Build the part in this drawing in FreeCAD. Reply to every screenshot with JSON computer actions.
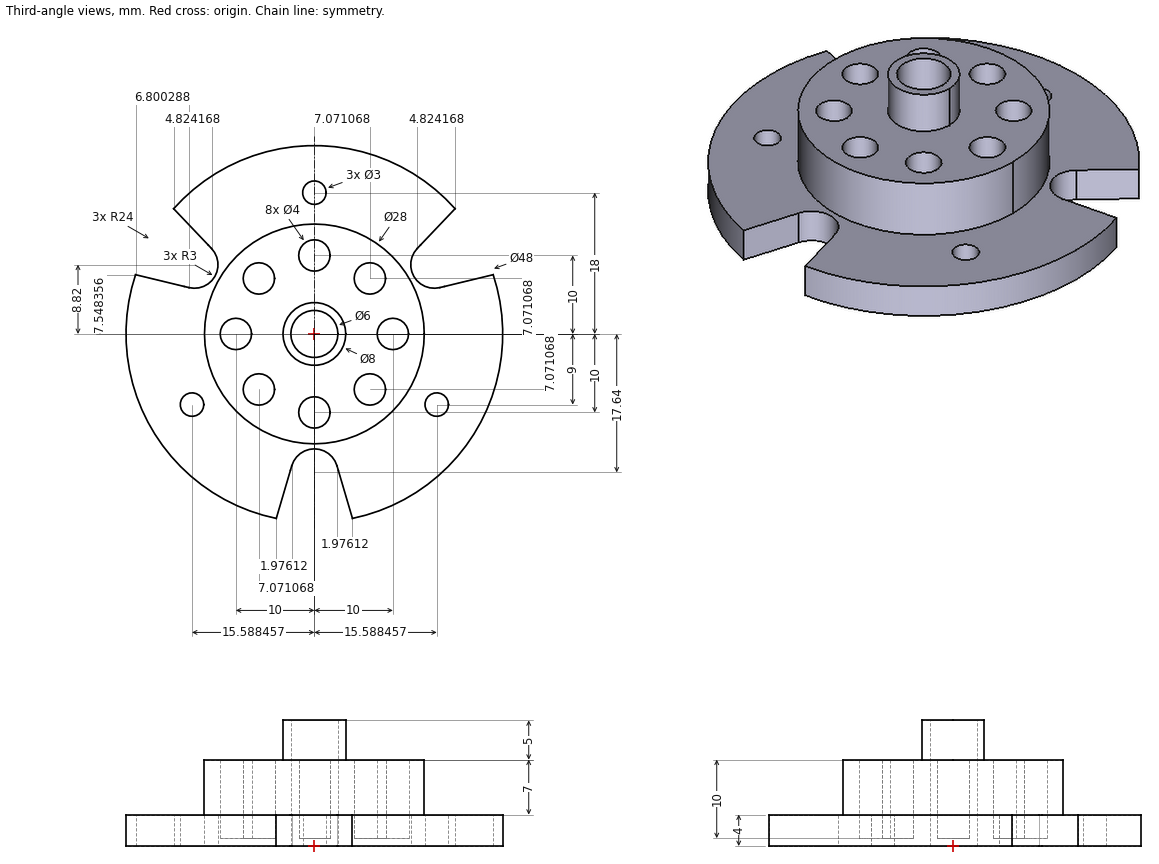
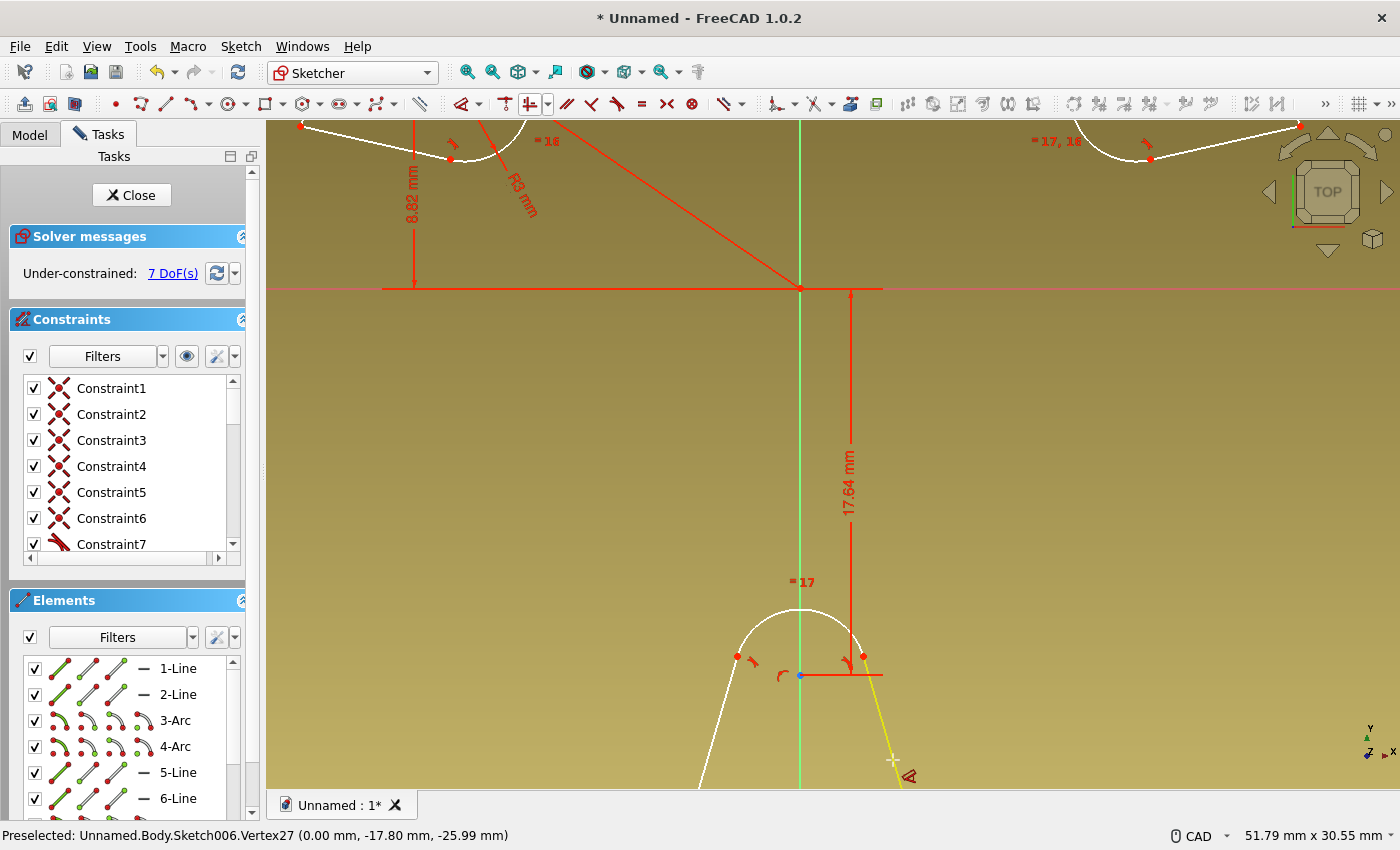
{"action": "left_click", "coordinate": [893, 760]}
{"action": "left_click", "coordinate": [885, 623]}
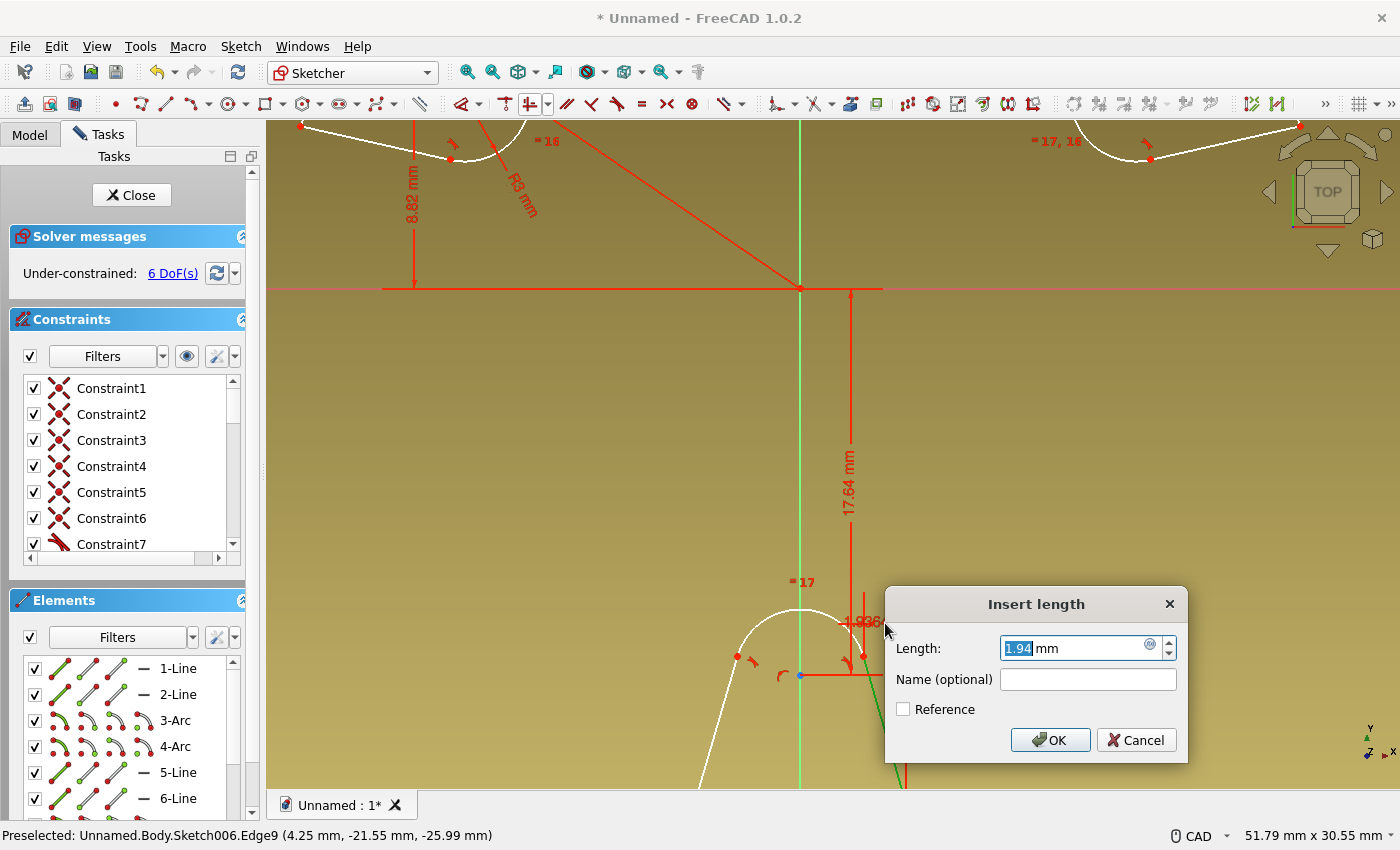
{"action": "type", "text": "1.97612"}
{"action": "key", "text": "Return"}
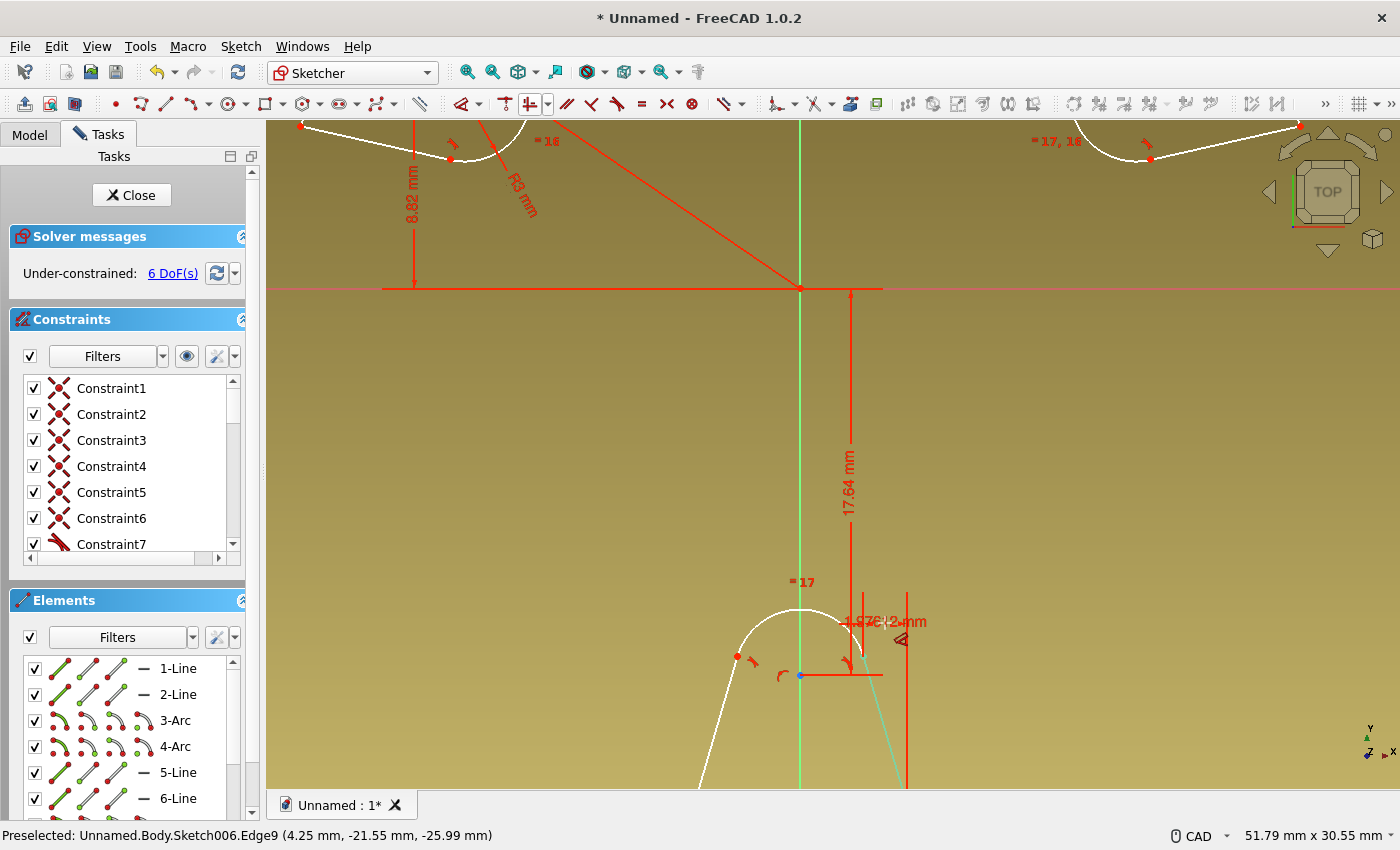
{"action": "left_click", "coordinate": [725, 701]}
{"action": "left_click", "coordinate": [716, 623]}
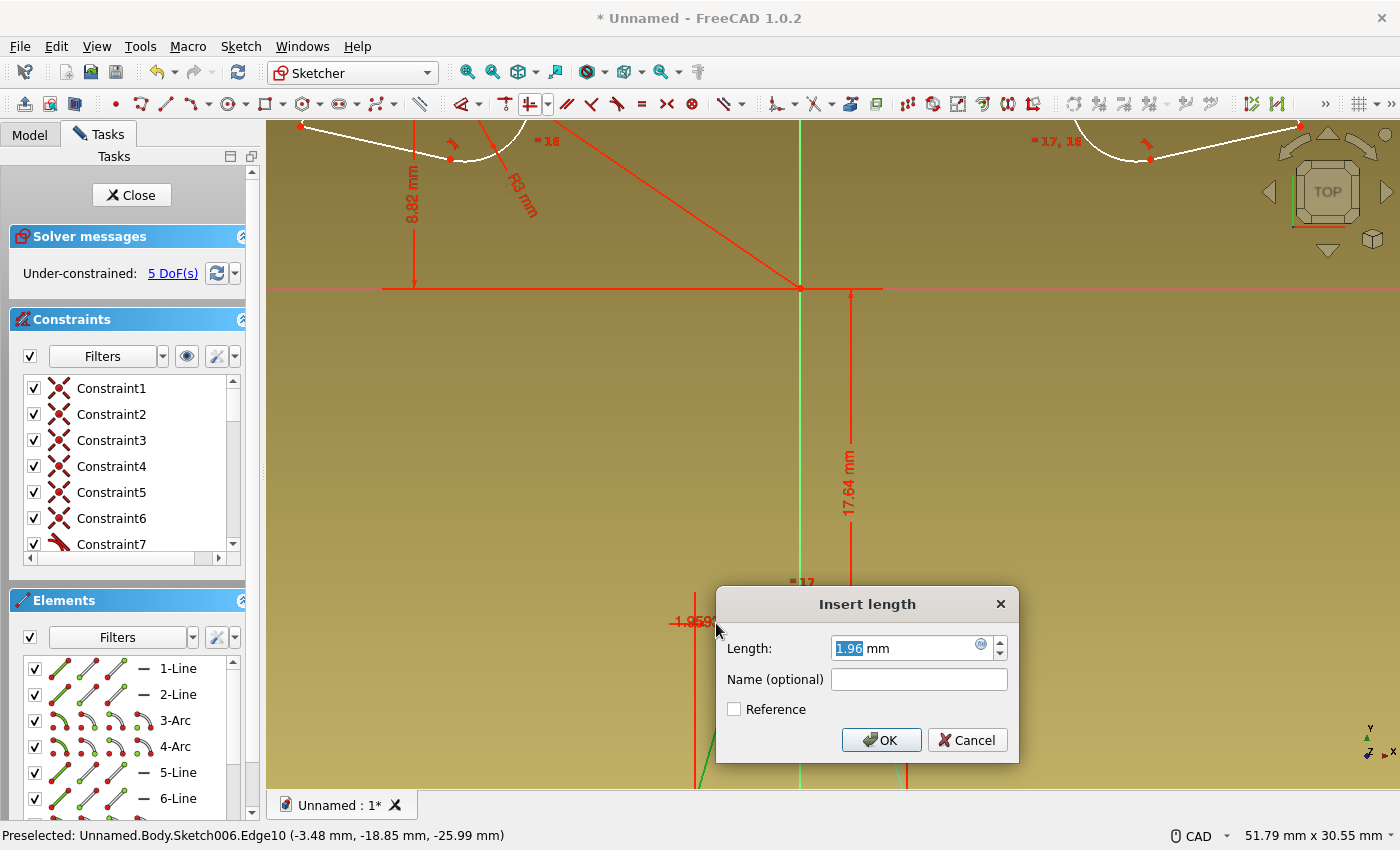
{"action": "type", "text": "1.97612"}
{"action": "key", "text": "Return"}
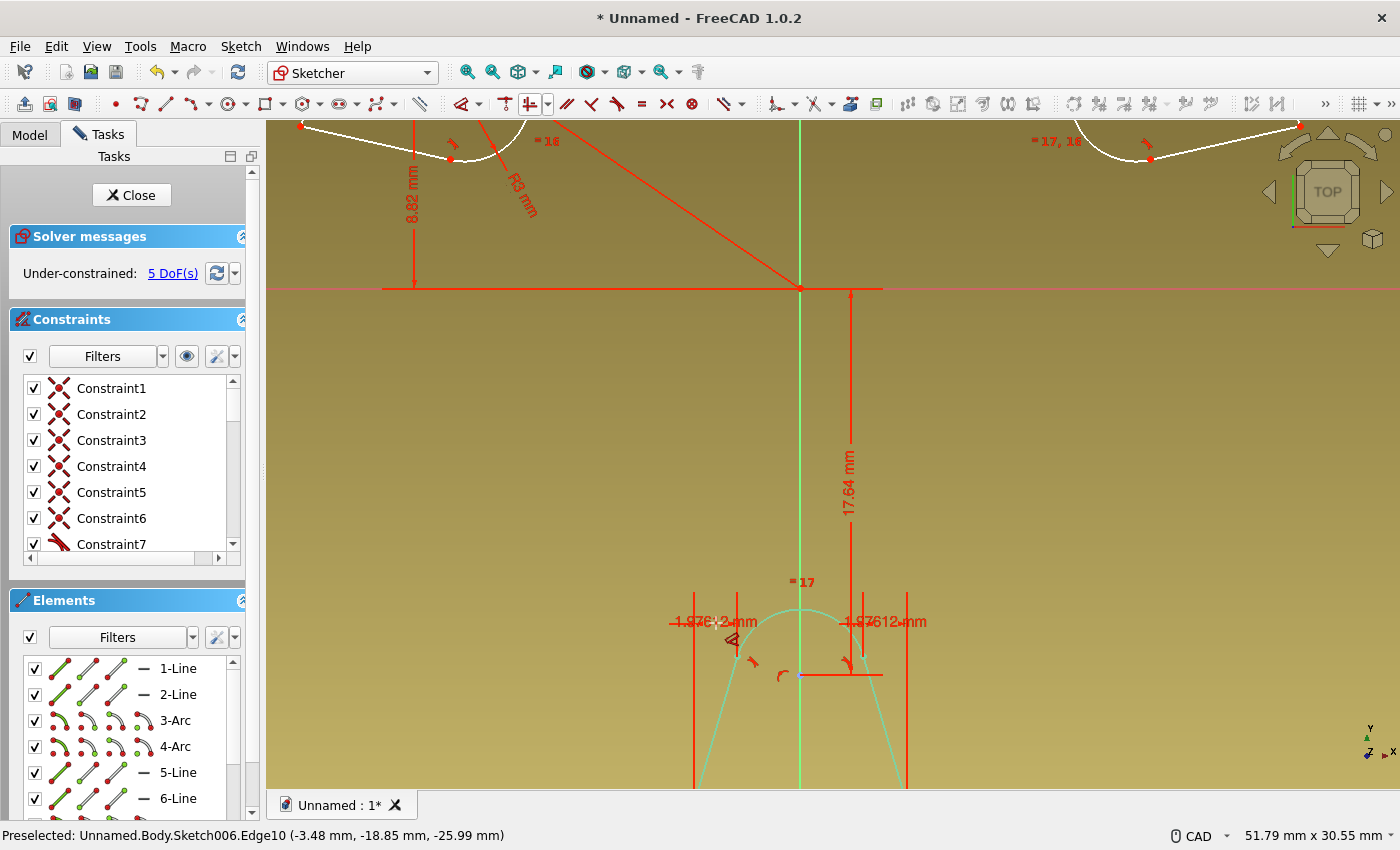
{"action": "scroll", "coordinate": [735, 518], "scroll_direction": "down", "scroll_amount": 4}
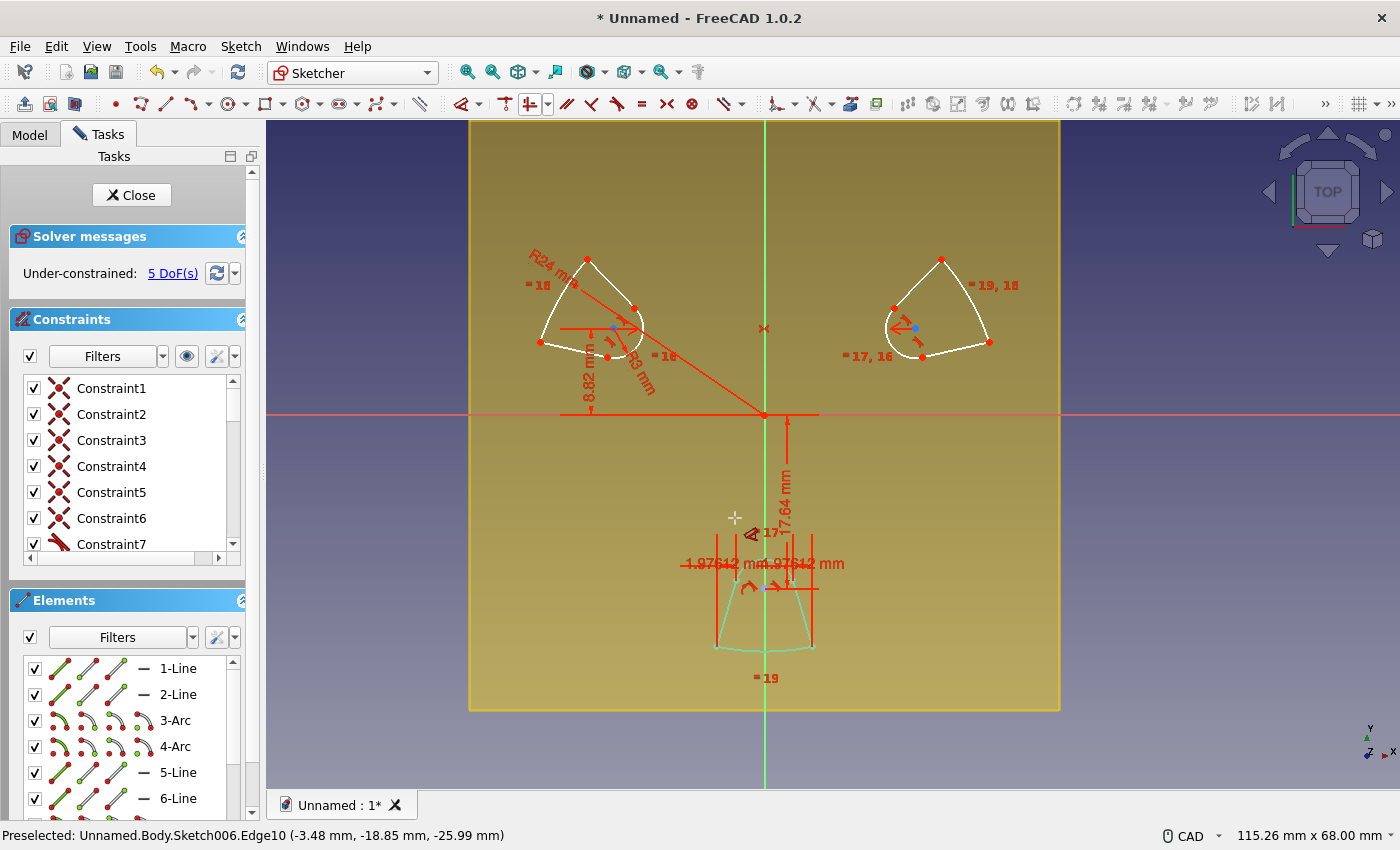
{"action": "left_click", "coordinate": [540, 342]}
{"action": "left_click", "coordinate": [506, 379]}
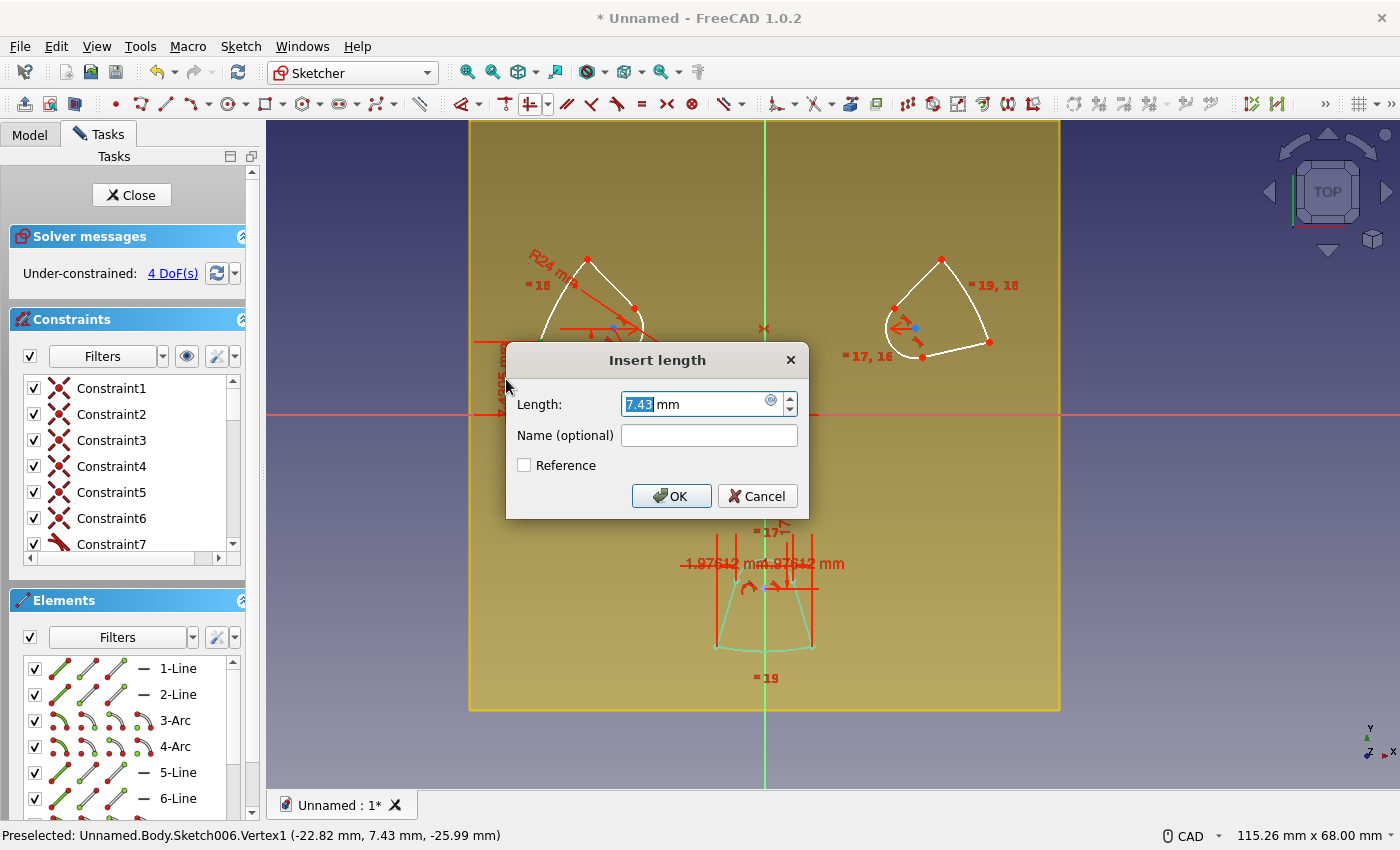
{"action": "type", "text": "7.548356"}
{"action": "key", "text": "Return"}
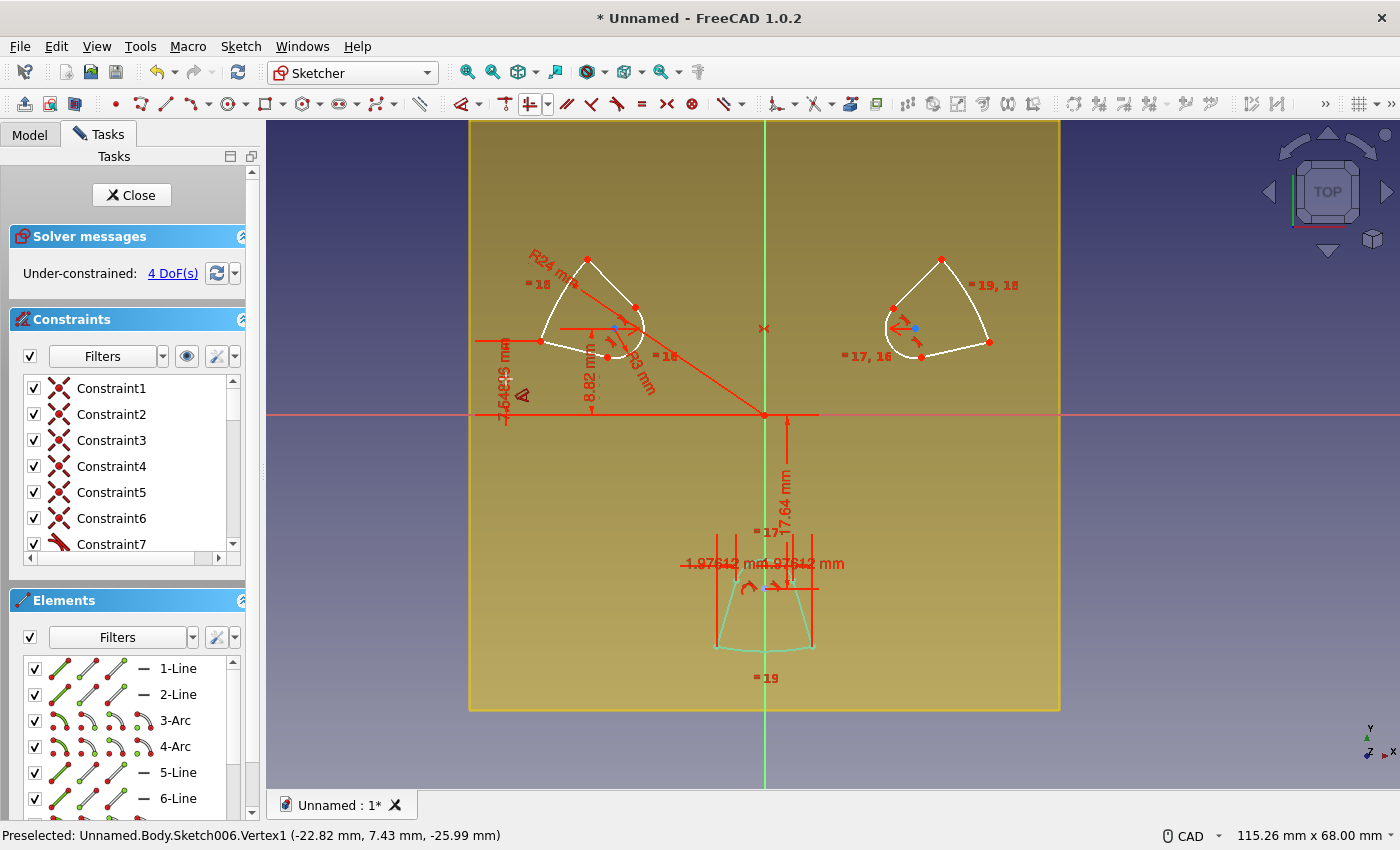
{"action": "left_click", "coordinate": [989, 342]}
{"action": "left_click", "coordinate": [1023, 379]}